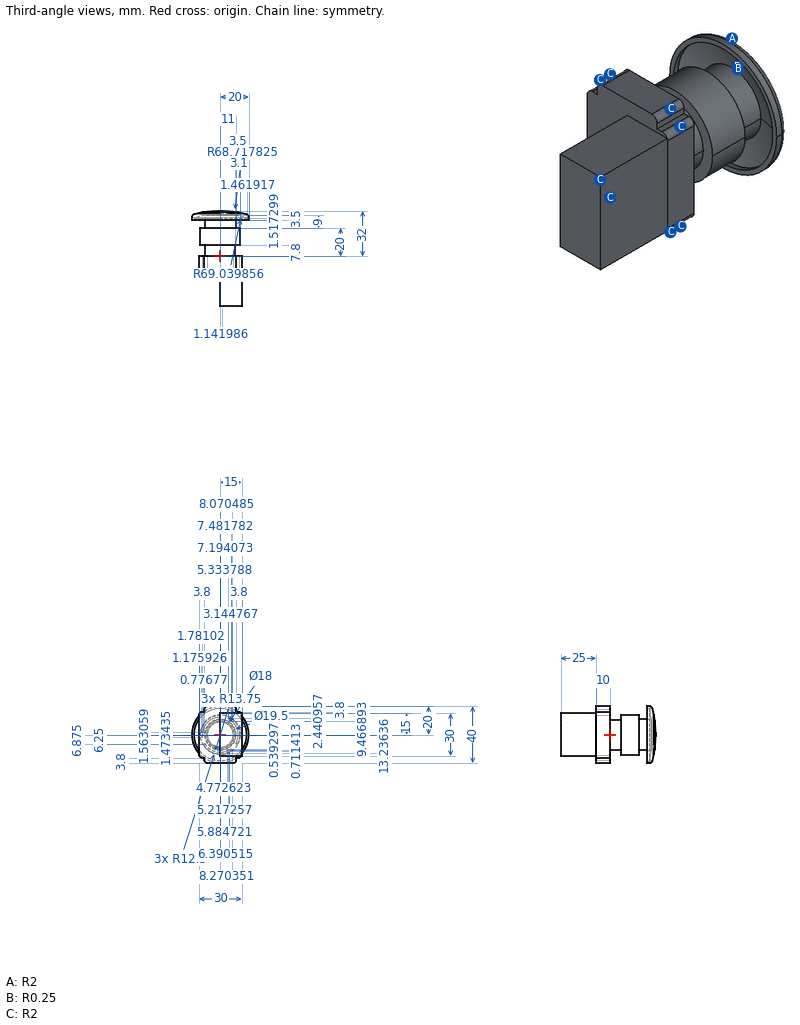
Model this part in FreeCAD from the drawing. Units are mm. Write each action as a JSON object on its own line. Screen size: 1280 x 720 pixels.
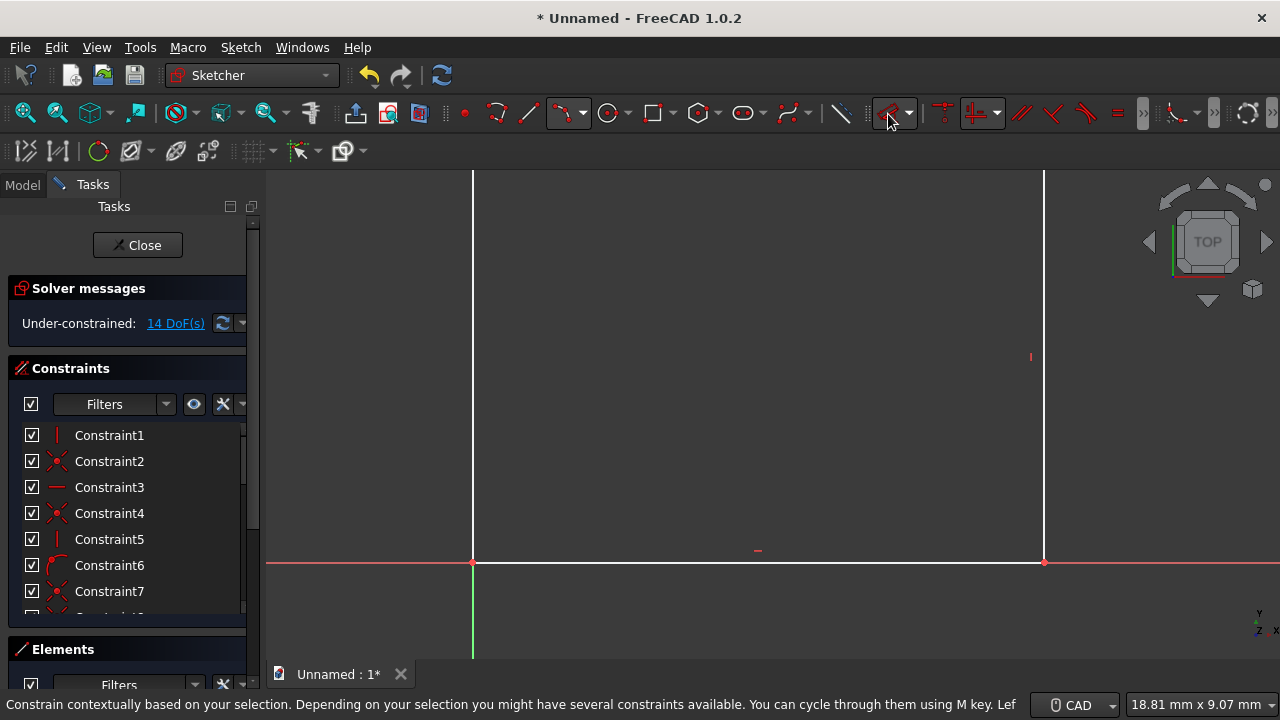
{"action": "scroll", "coordinate": [644, 556], "scroll_direction": "down", "scroll_amount": 9}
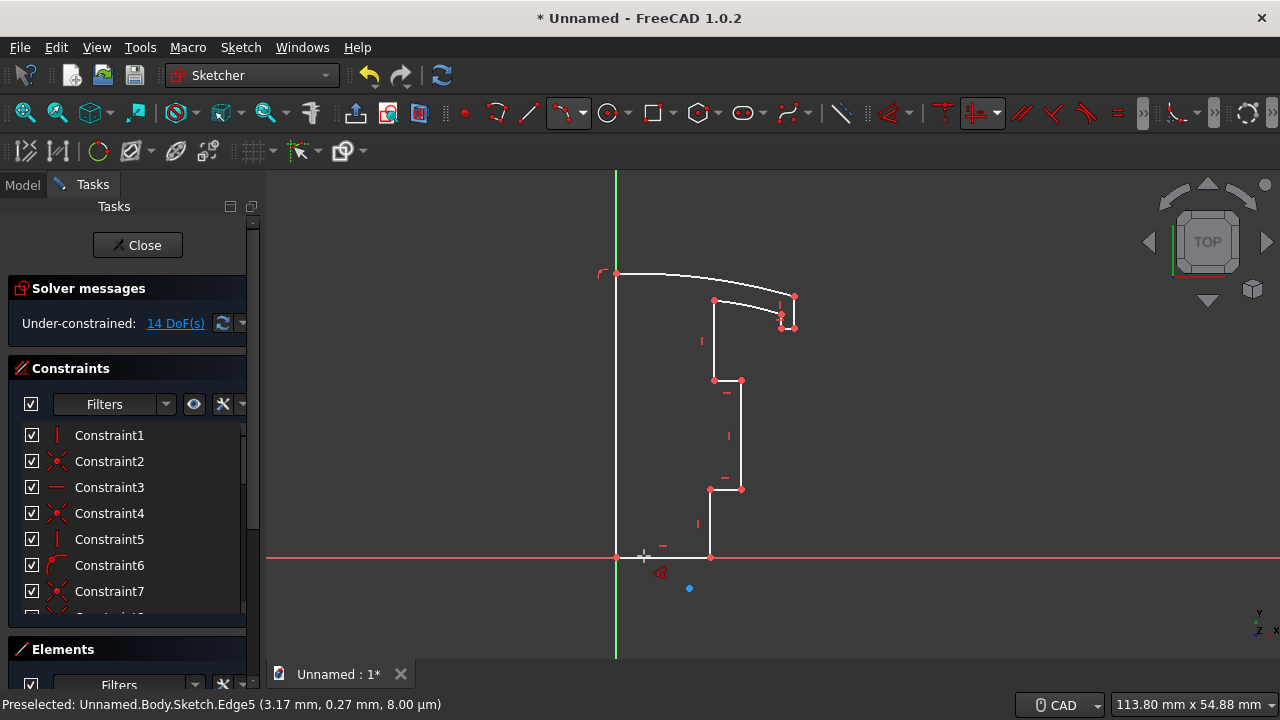
{"action": "left_click", "coordinate": [742, 284]}
{"action": "left_click", "coordinate": [748, 253]}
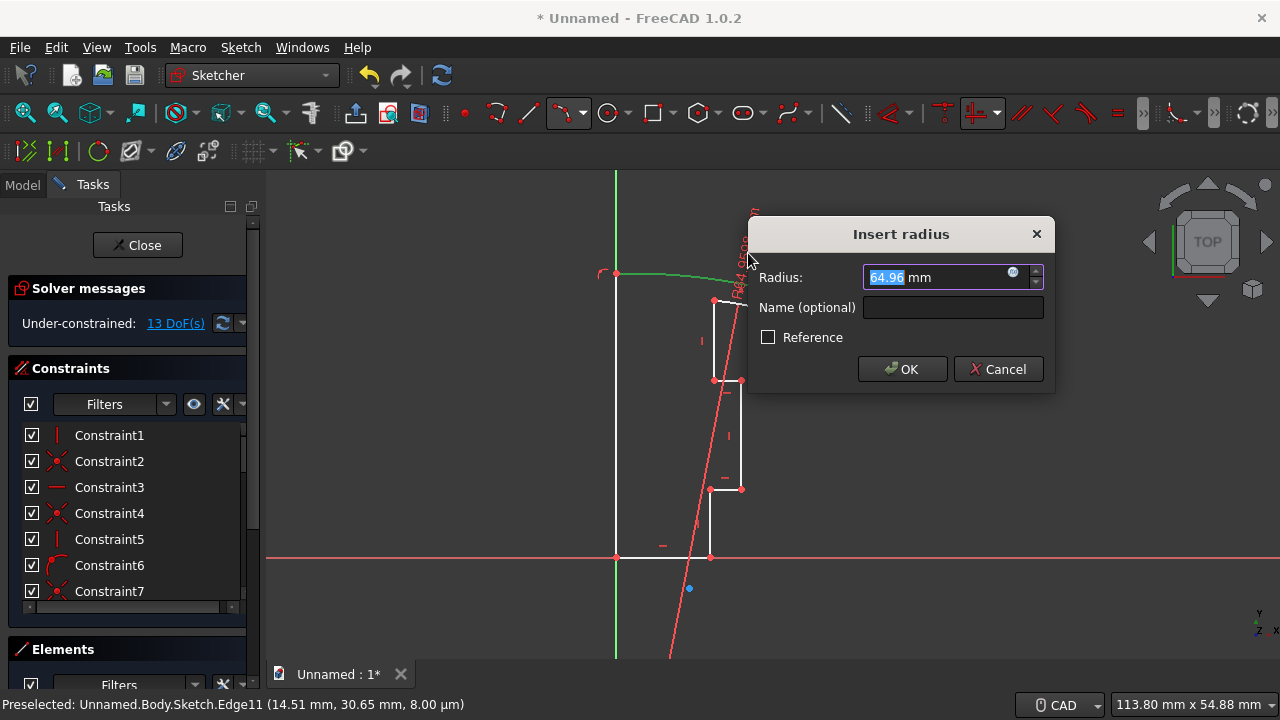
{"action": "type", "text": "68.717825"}
{"action": "key", "text": "Return"}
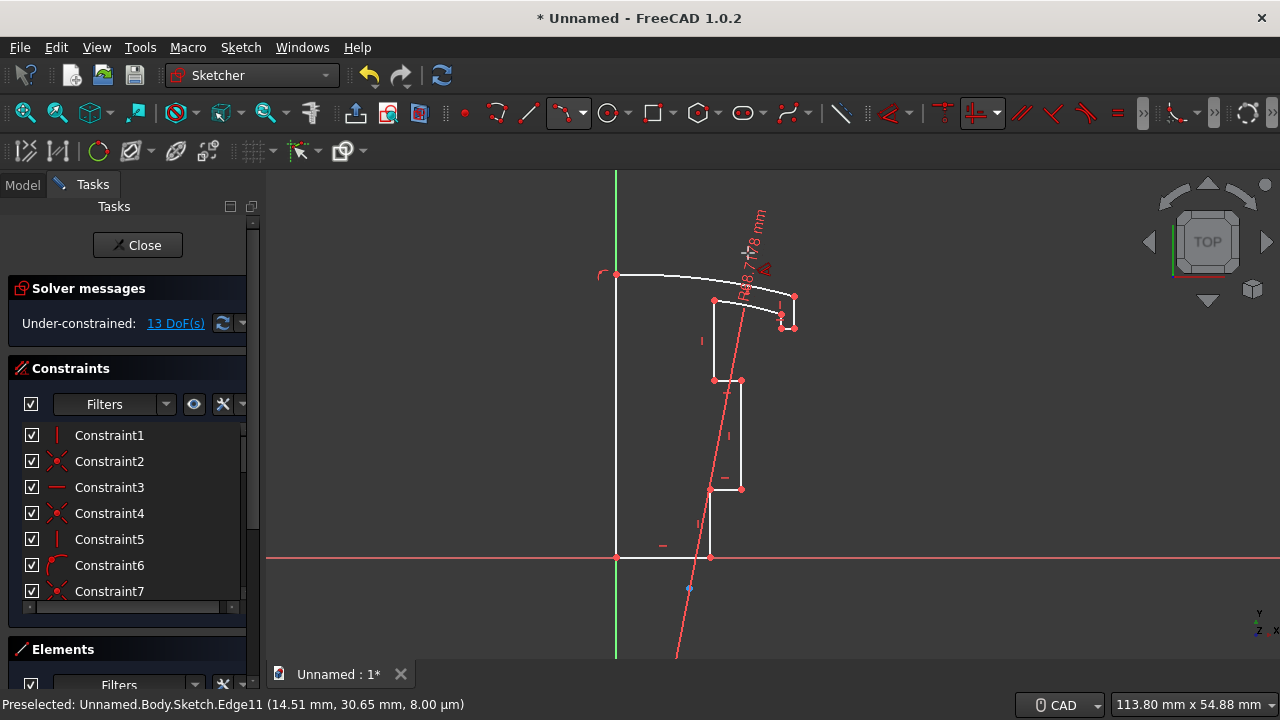
{"action": "left_click", "coordinate": [762, 309]}
{"action": "left_click", "coordinate": [909, 355]}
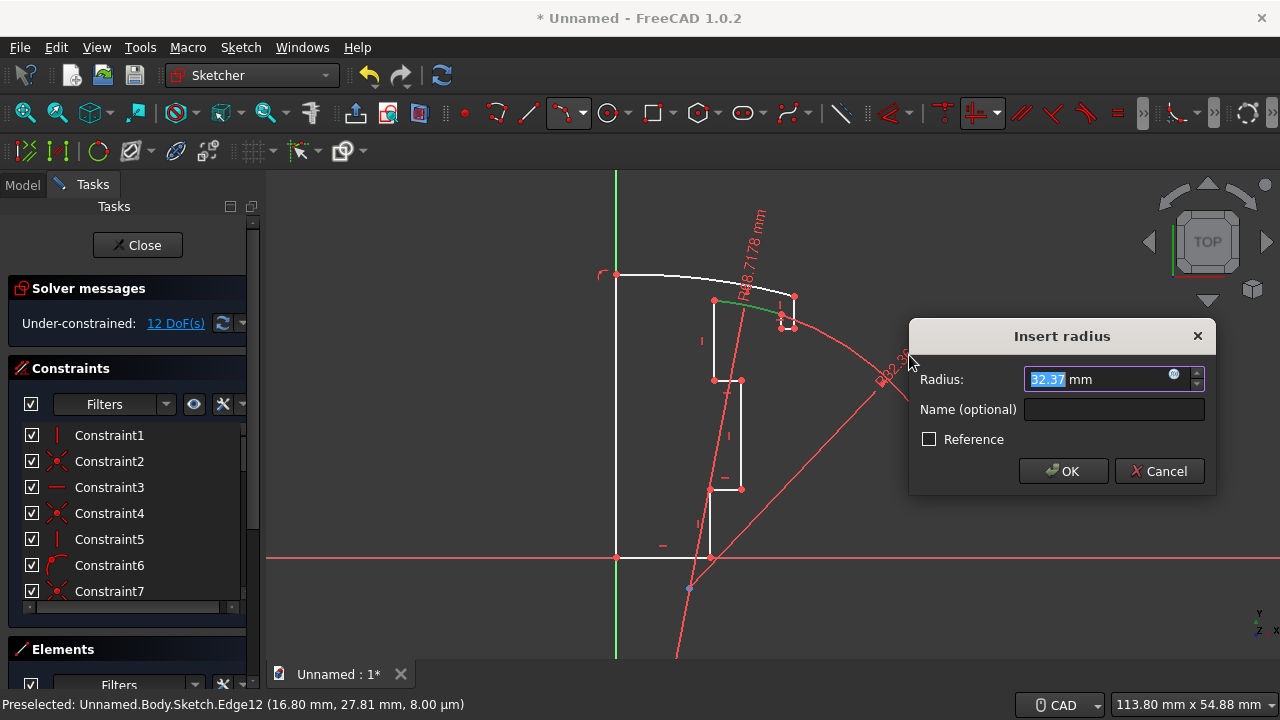
{"action": "type", "text": "69.039856"}
{"action": "key", "text": "Return"}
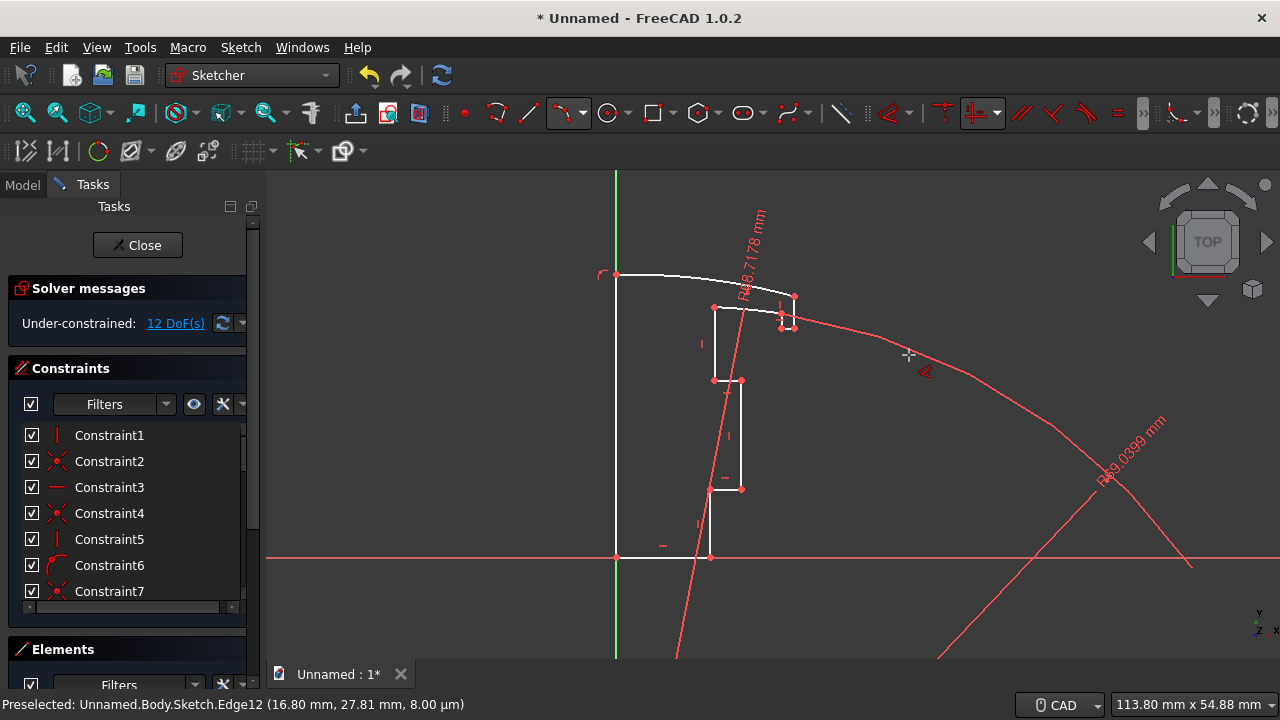
{"action": "left_click", "coordinate": [715, 359]}
{"action": "left_click", "coordinate": [749, 344]}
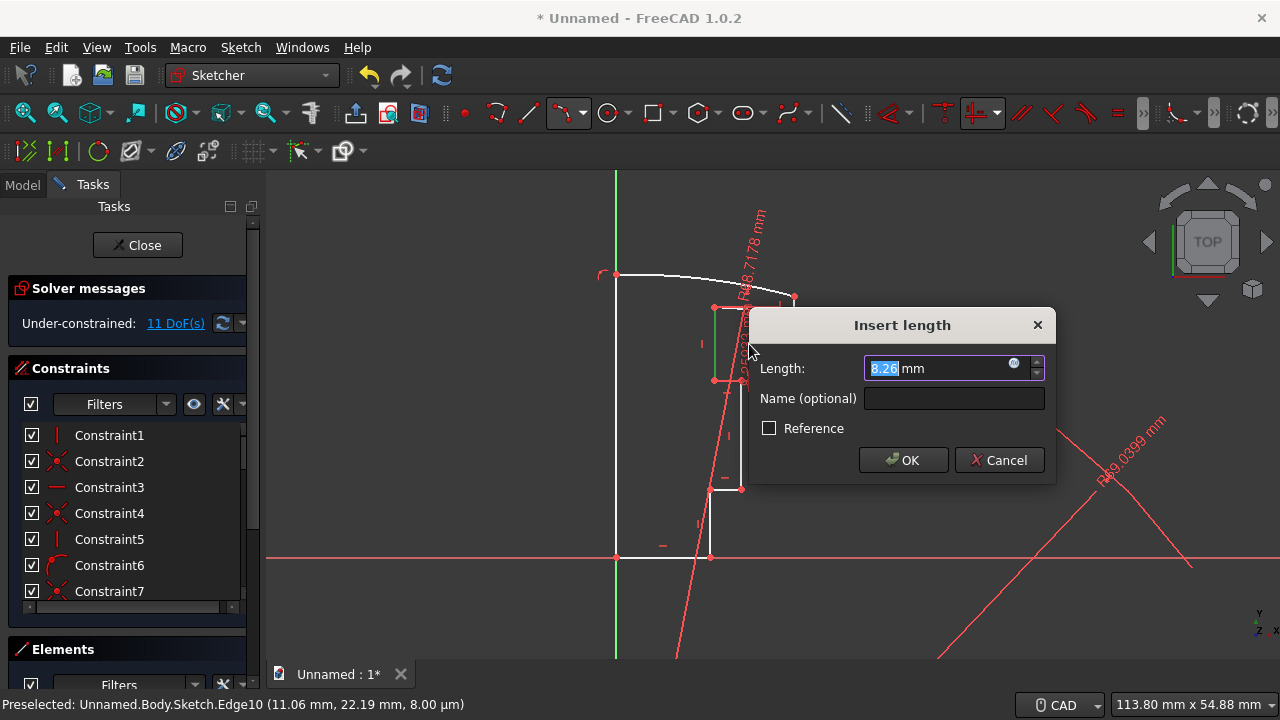
{"action": "type", "text": "9"}
{"action": "key", "text": "Return"}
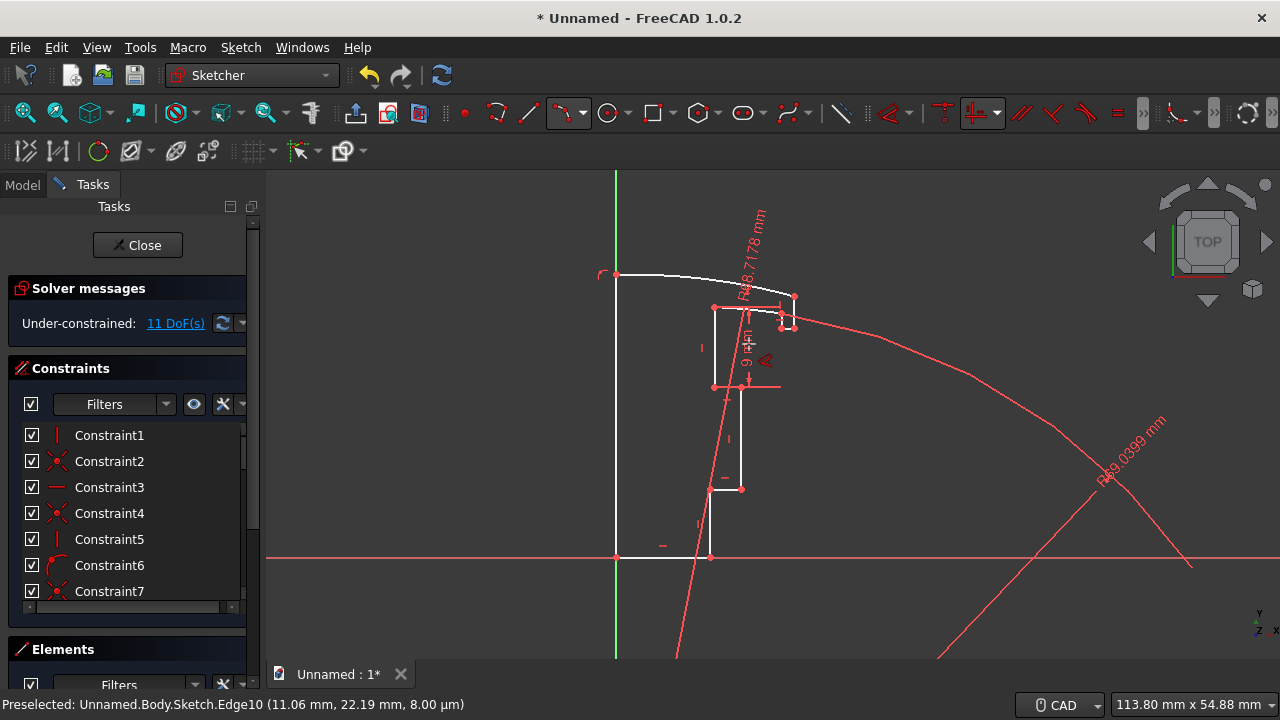
{"action": "left_click", "coordinate": [616, 360]}
{"action": "left_click", "coordinate": [582, 416]}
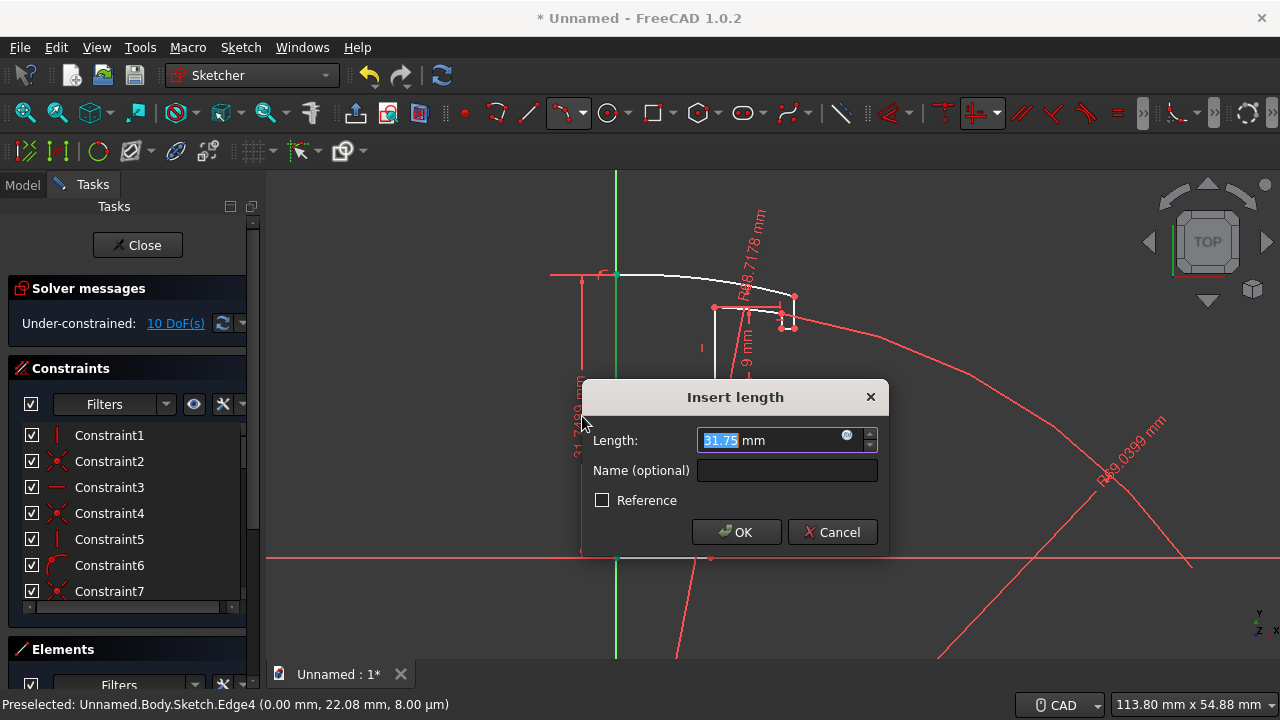
{"action": "type", "text": "32"}
{"action": "key", "text": "Return"}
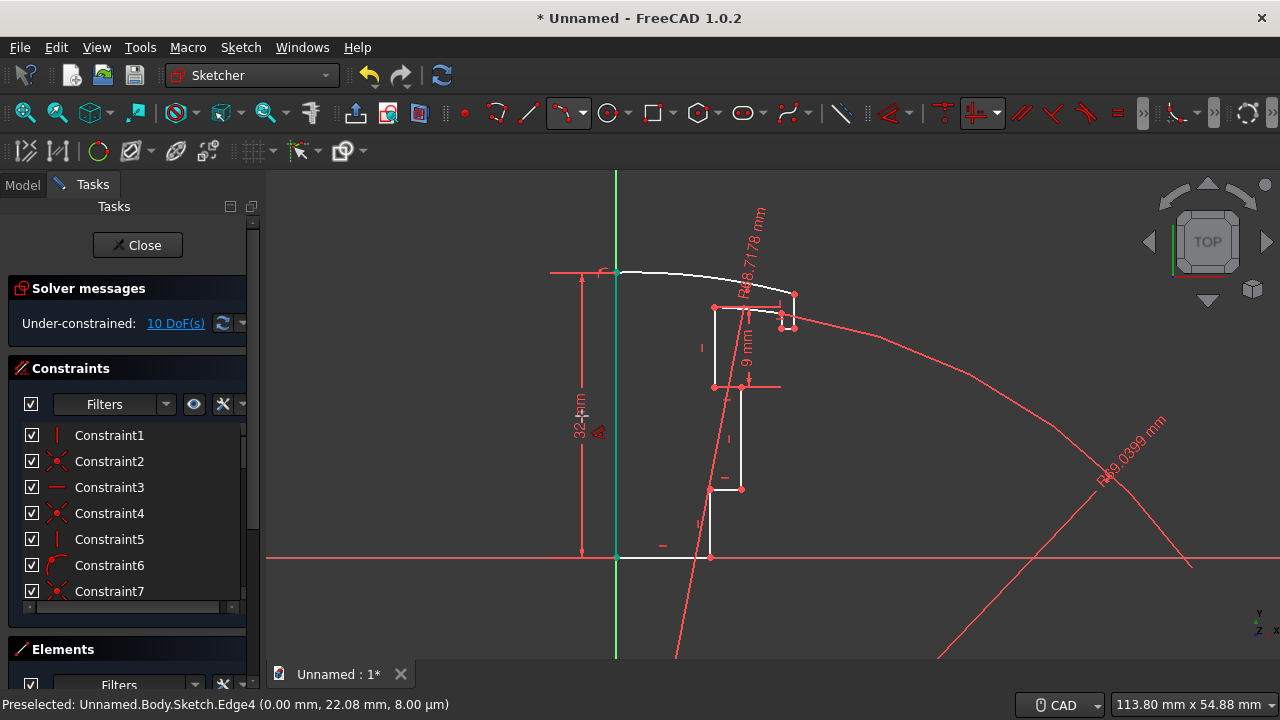
{"action": "scroll", "coordinate": [794, 318], "scroll_direction": "up", "scroll_amount": 2}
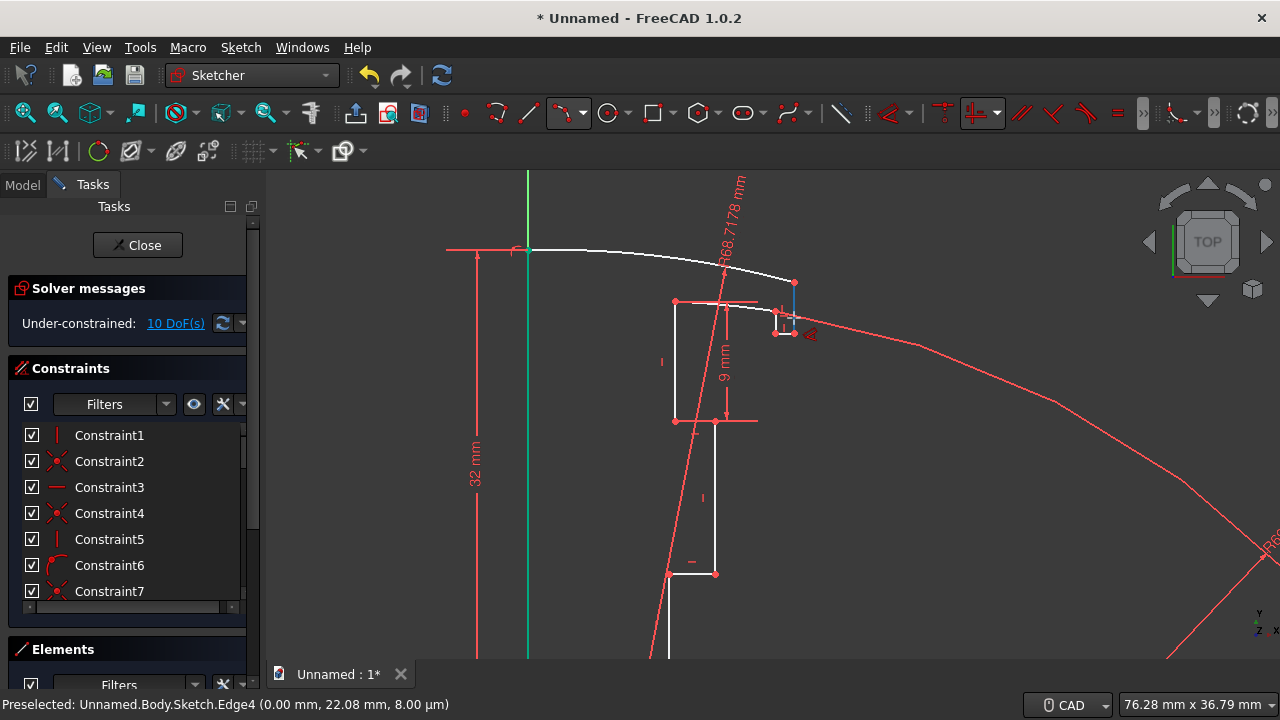
{"action": "left_click", "coordinate": [794, 318]}
{"action": "left_click", "coordinate": [828, 308]}